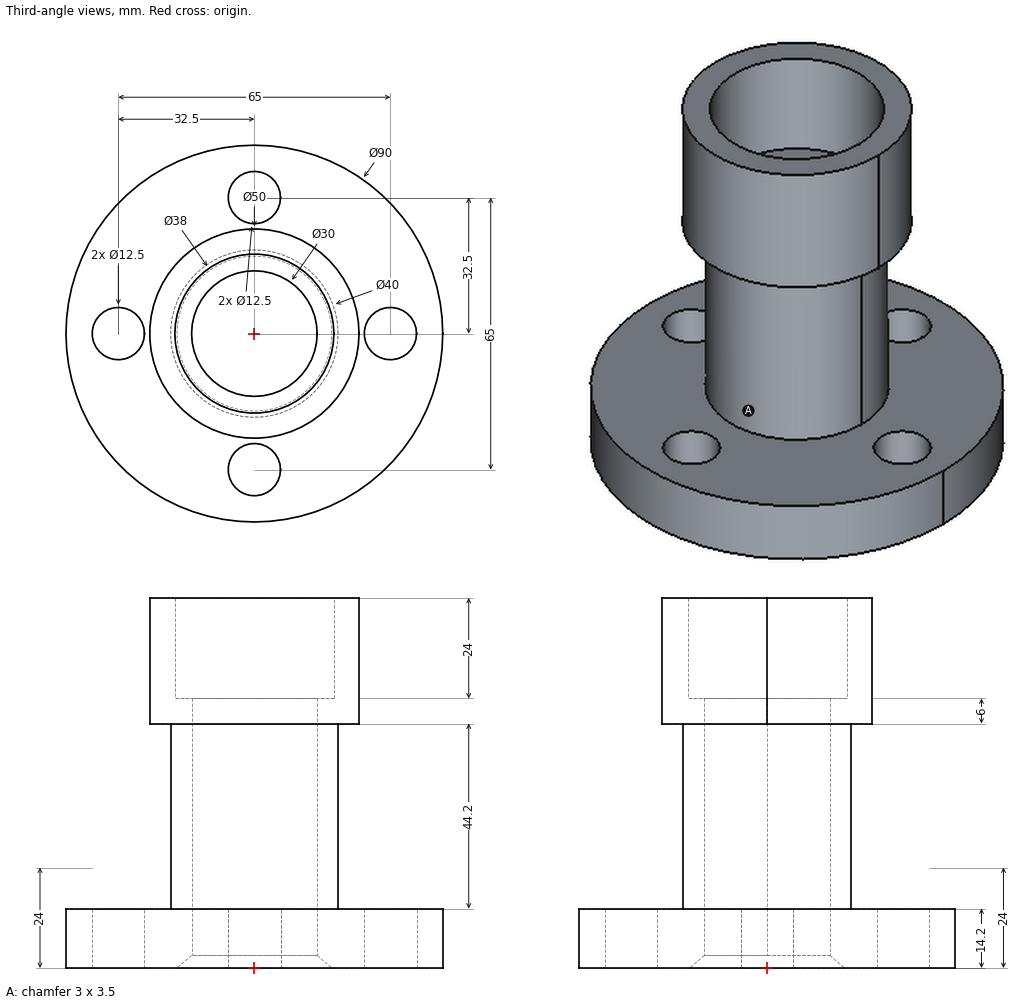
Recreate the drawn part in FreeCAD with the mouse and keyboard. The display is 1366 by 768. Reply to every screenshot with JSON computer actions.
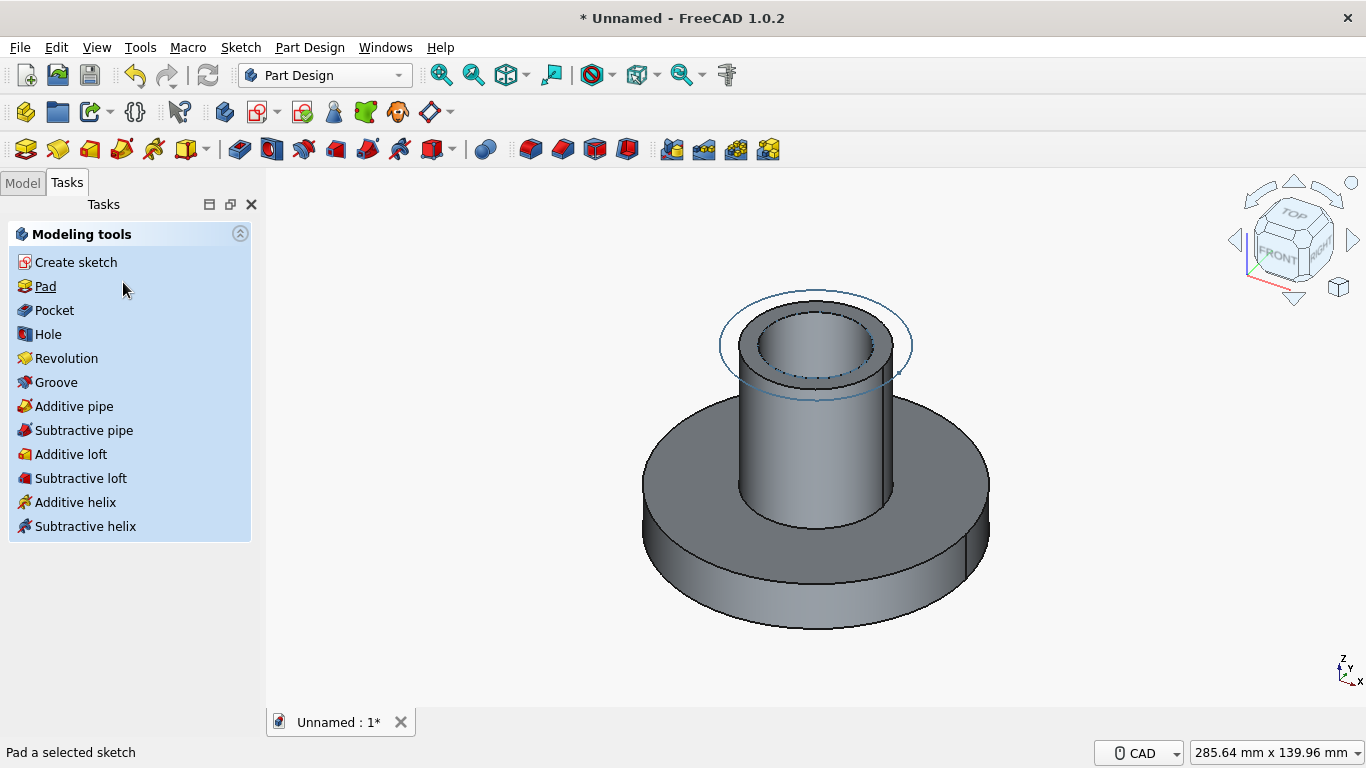
{"action": "left_click", "coordinate": [26, 150]}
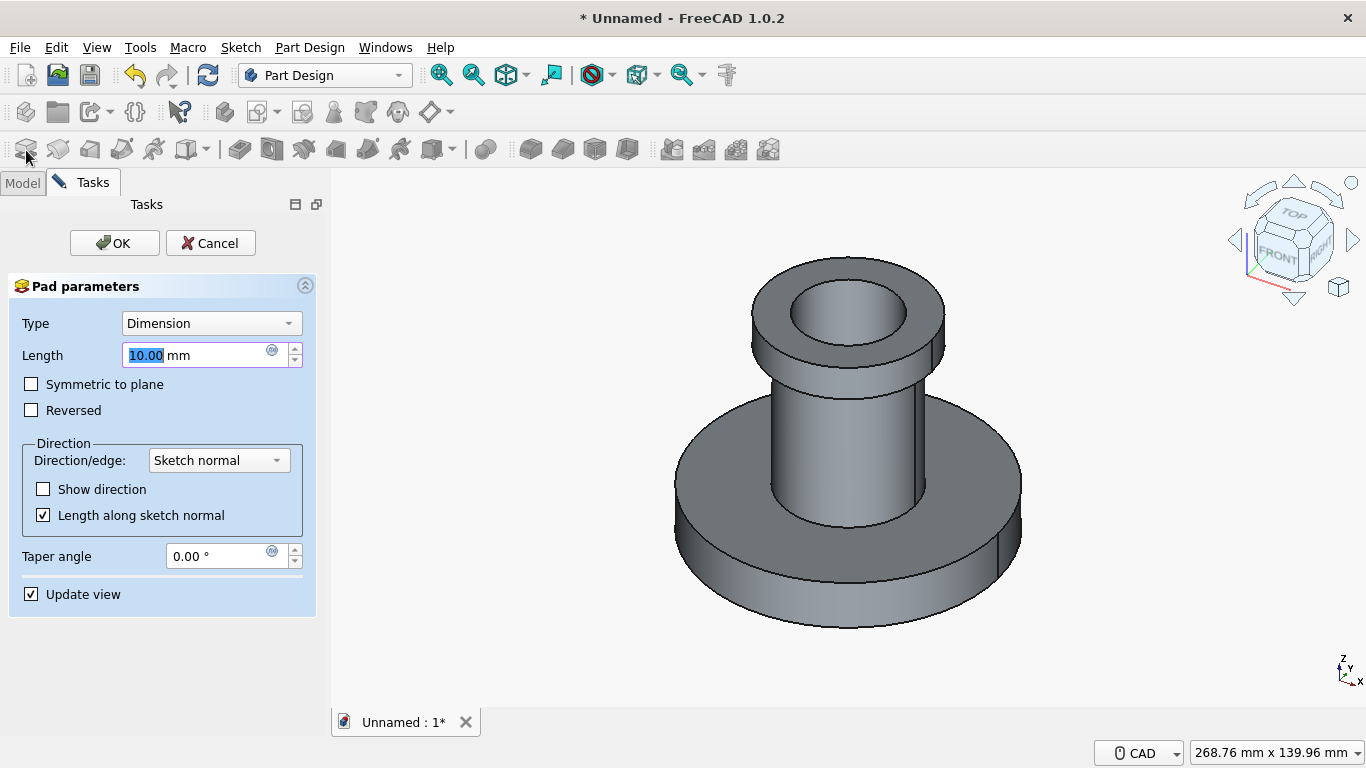
{"action": "type", "text": "6"}
{"action": "key", "text": "Tab"}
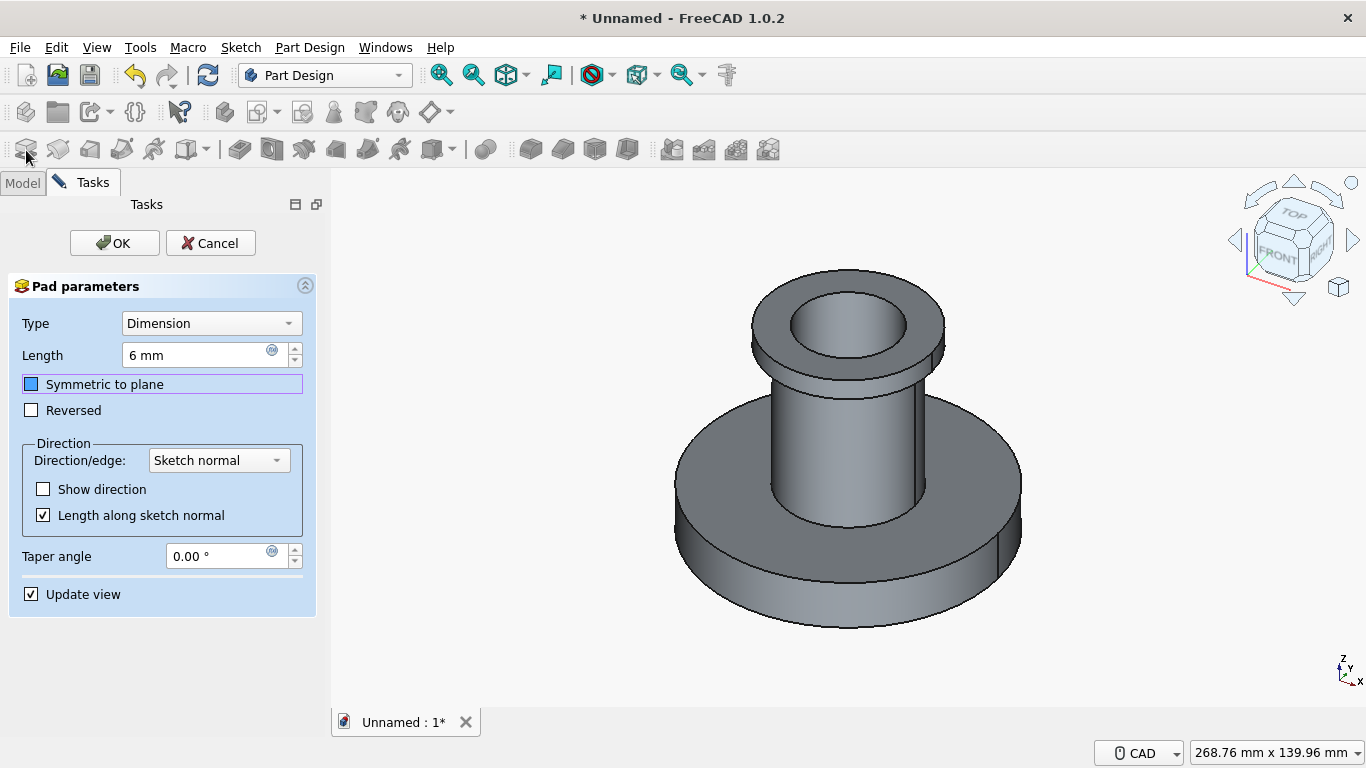
{"action": "left_click", "coordinate": [115, 243]}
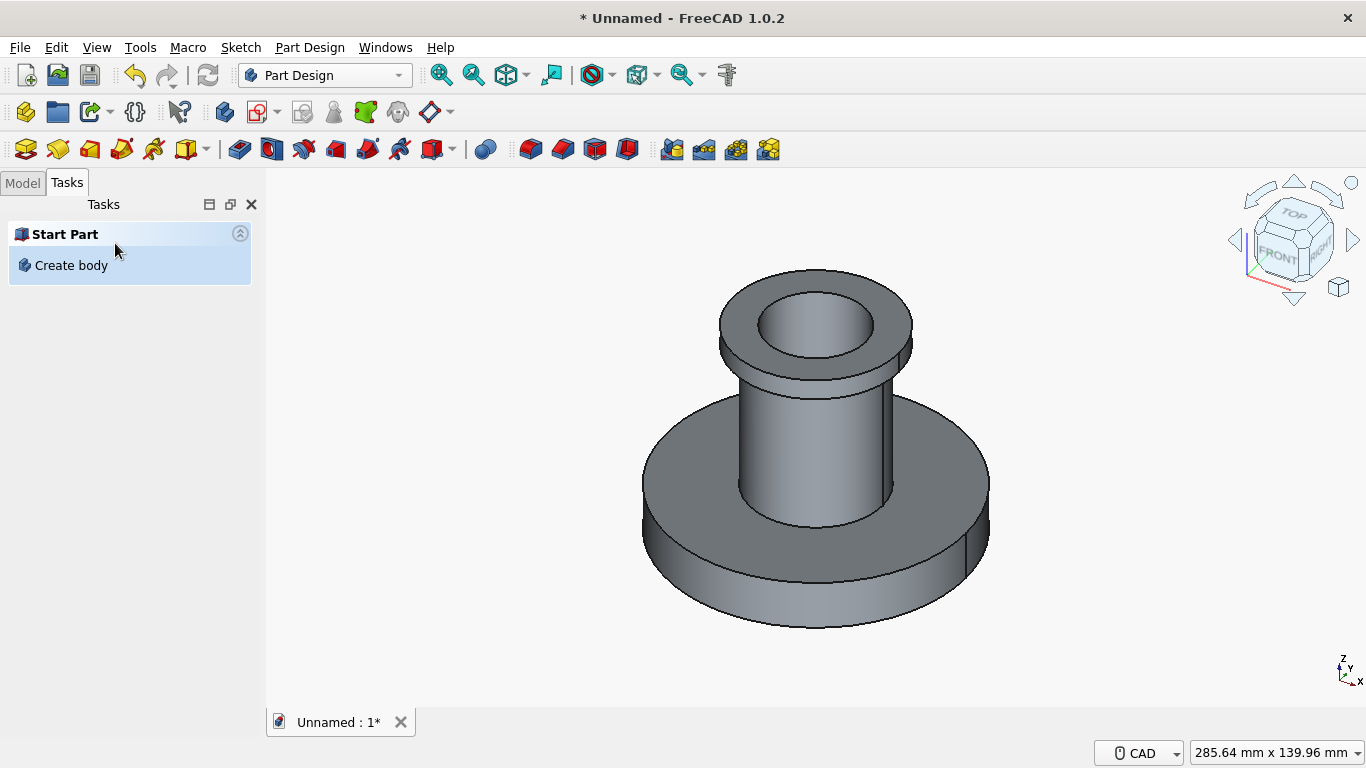
{"action": "left_click", "coordinate": [836, 367]}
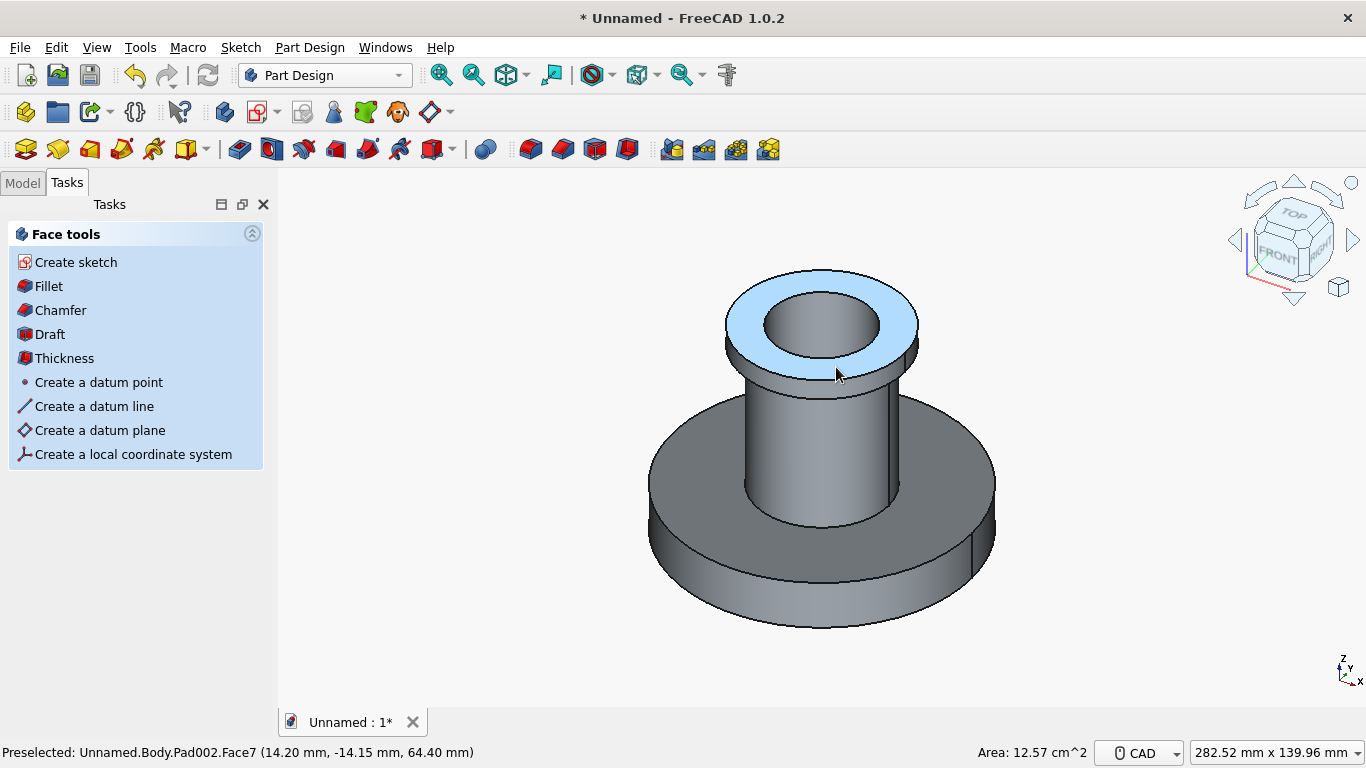
{"action": "left_click", "coordinate": [258, 112]}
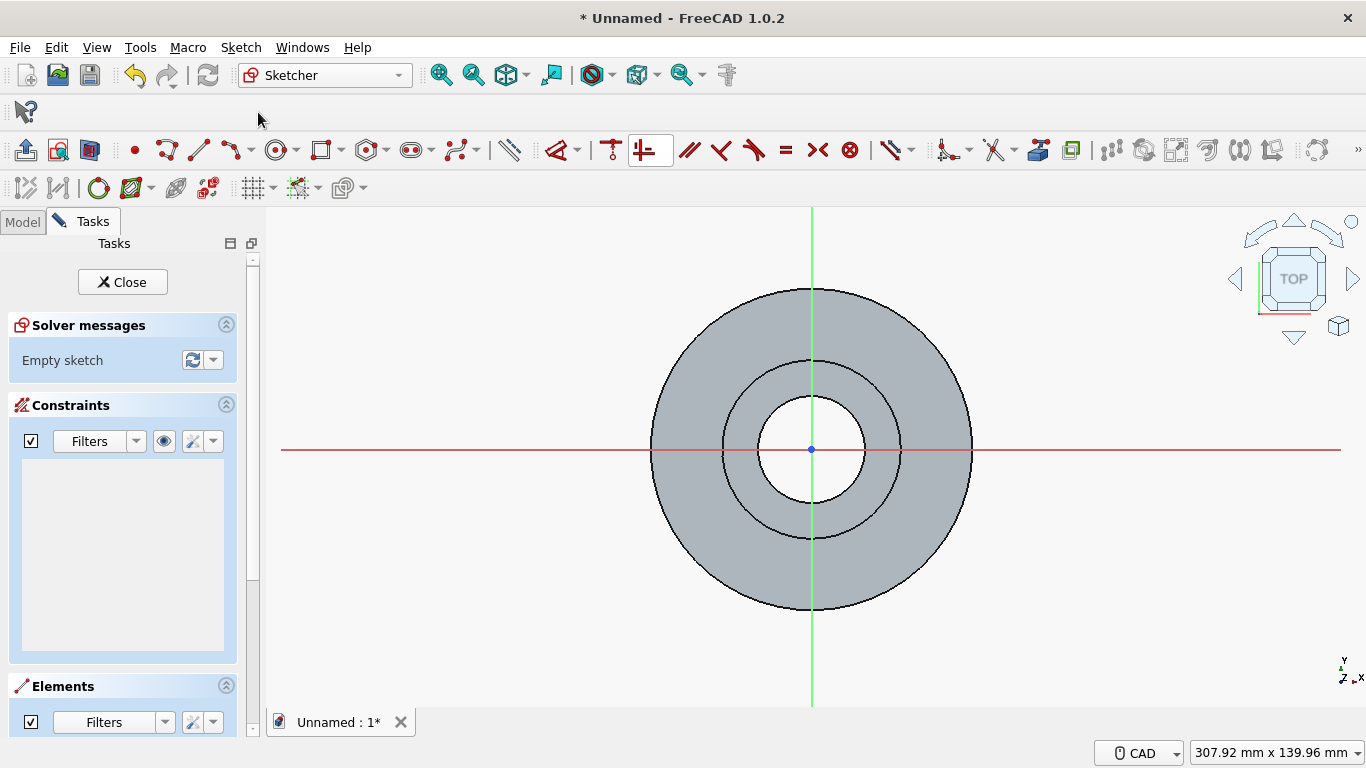
{"action": "scroll", "coordinate": [889, 440], "scroll_direction": "up", "scroll_amount": 3}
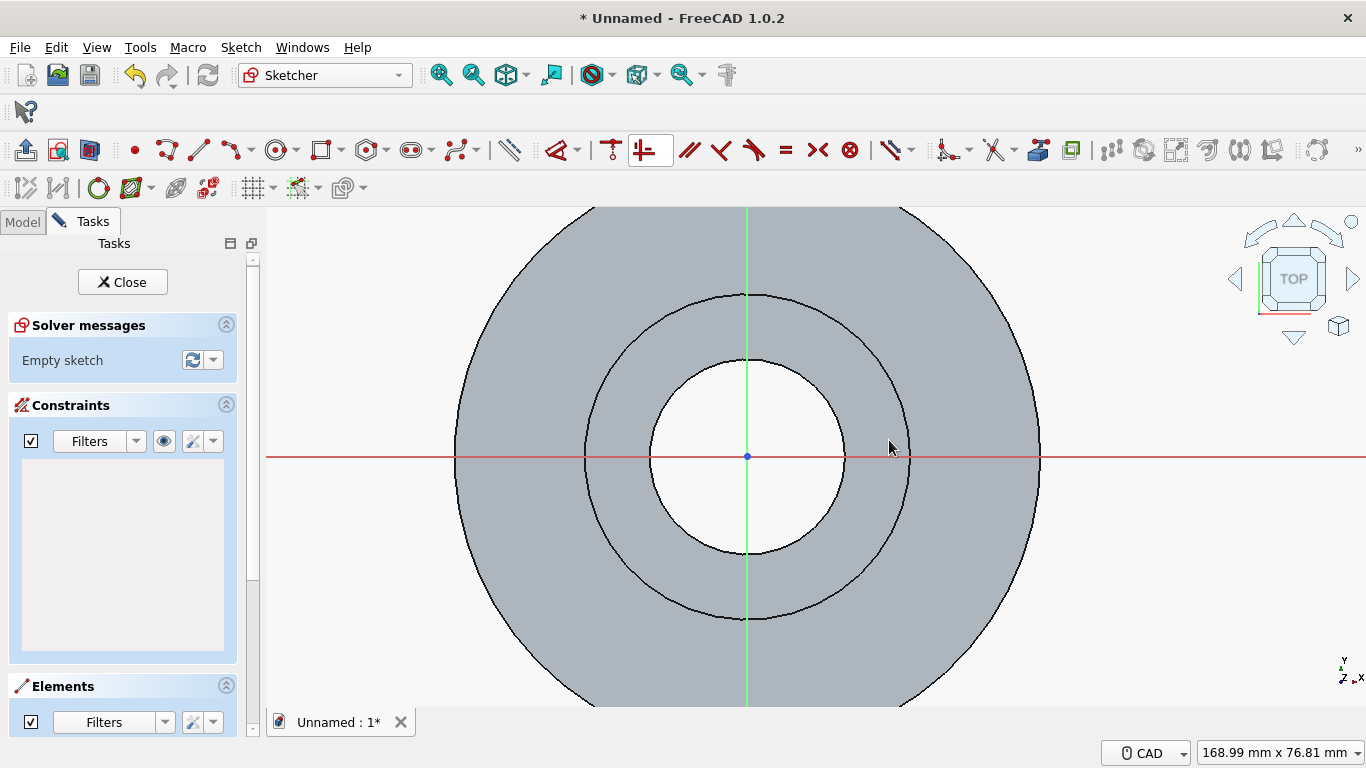
{"action": "left_click", "coordinate": [276, 150]}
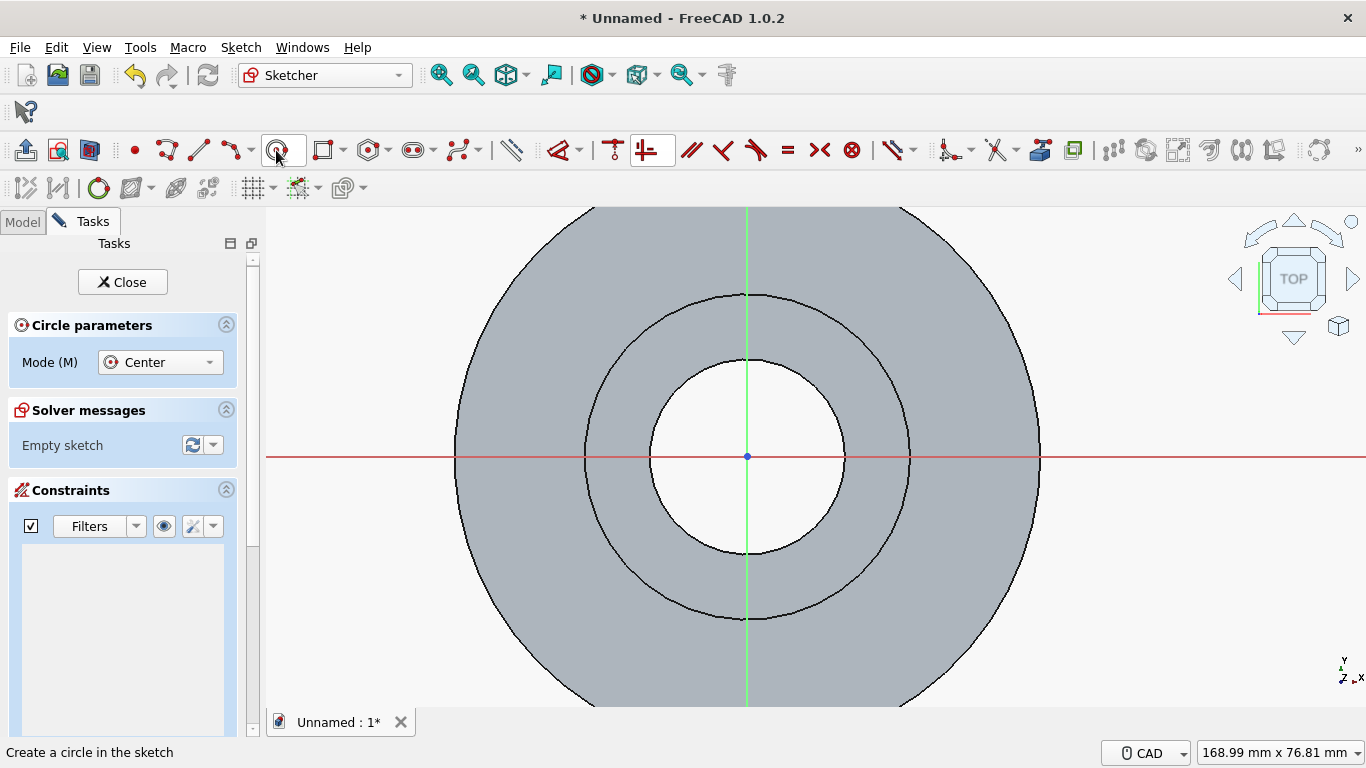
{"action": "left_click", "coordinate": [747, 457]}
{"action": "mouse_move", "coordinate": [862, 342]}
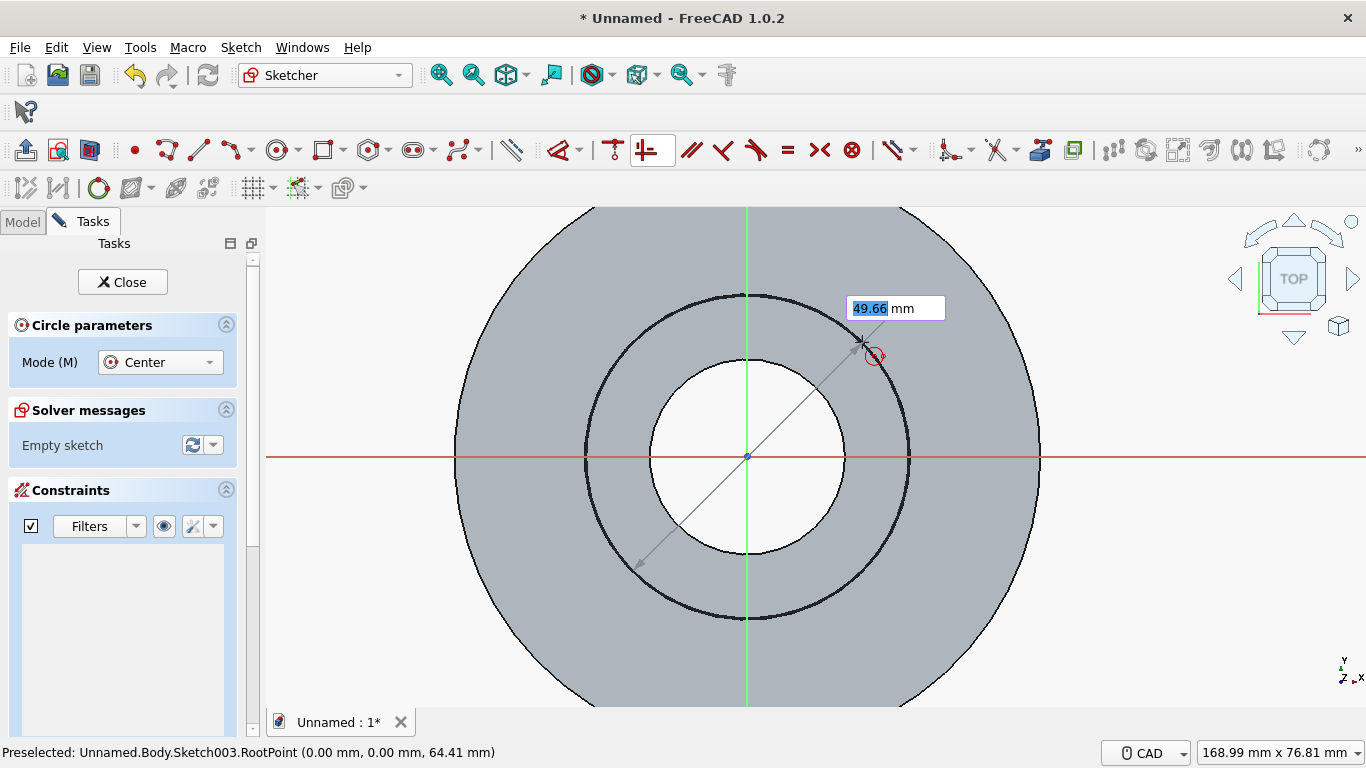
{"action": "type", "text": "50"}
{"action": "key", "text": "Return"}